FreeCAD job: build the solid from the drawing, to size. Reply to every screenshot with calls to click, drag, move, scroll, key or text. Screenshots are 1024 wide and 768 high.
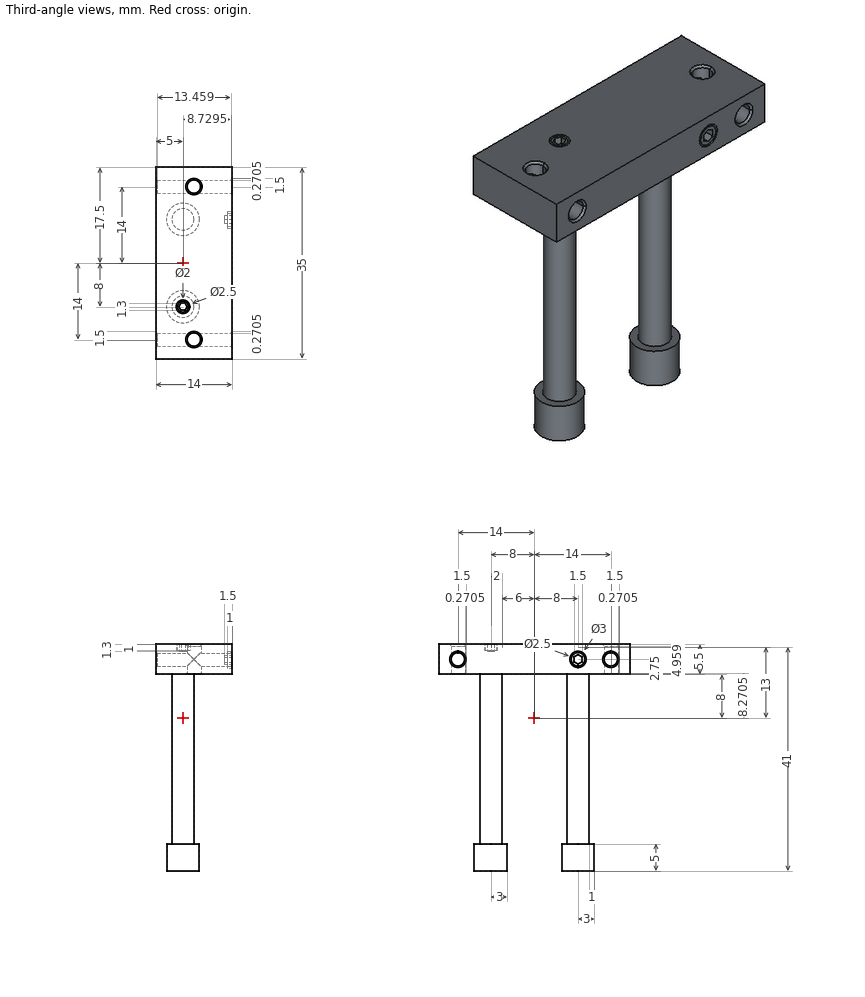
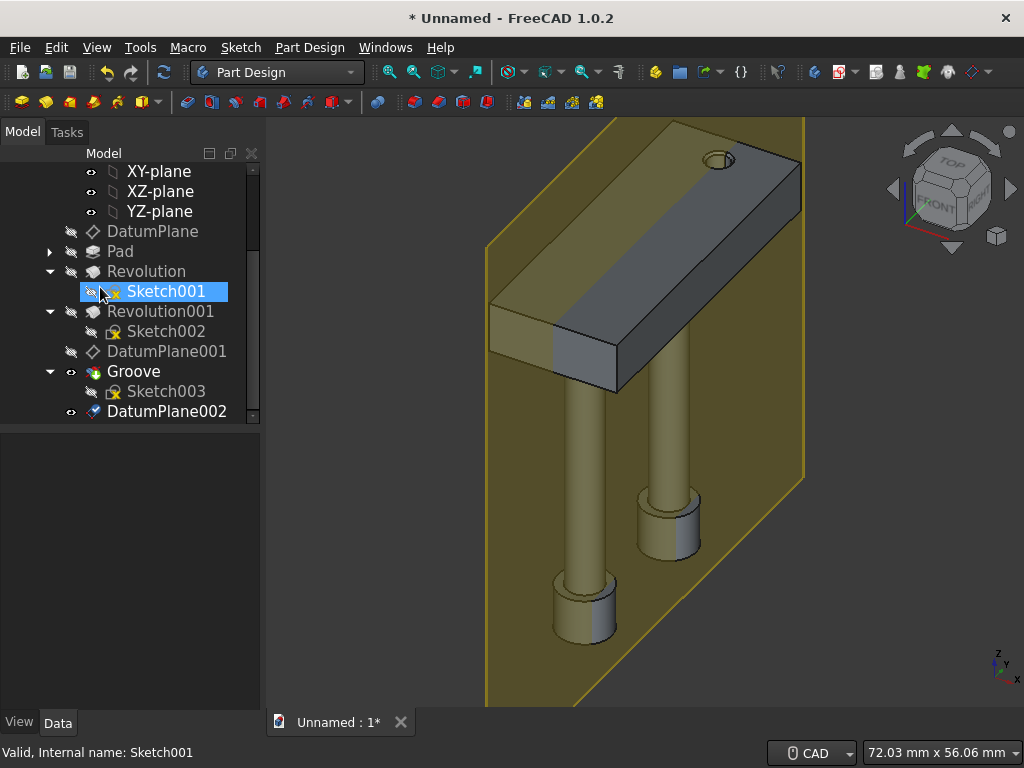
click(116, 412)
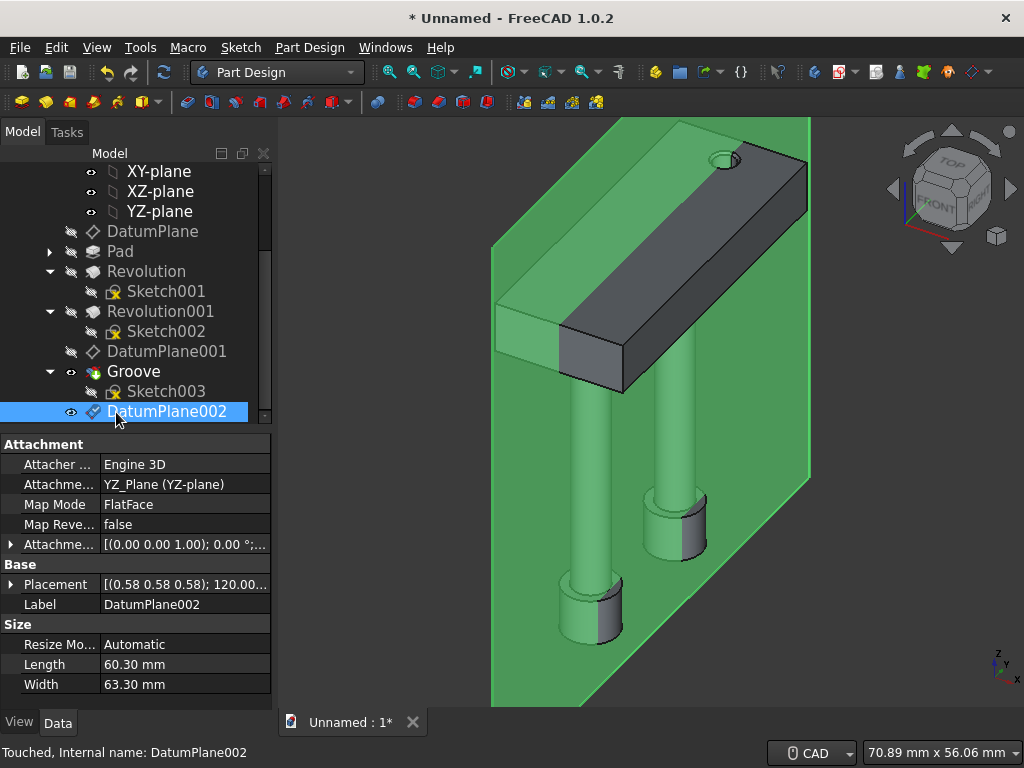
click(840, 72)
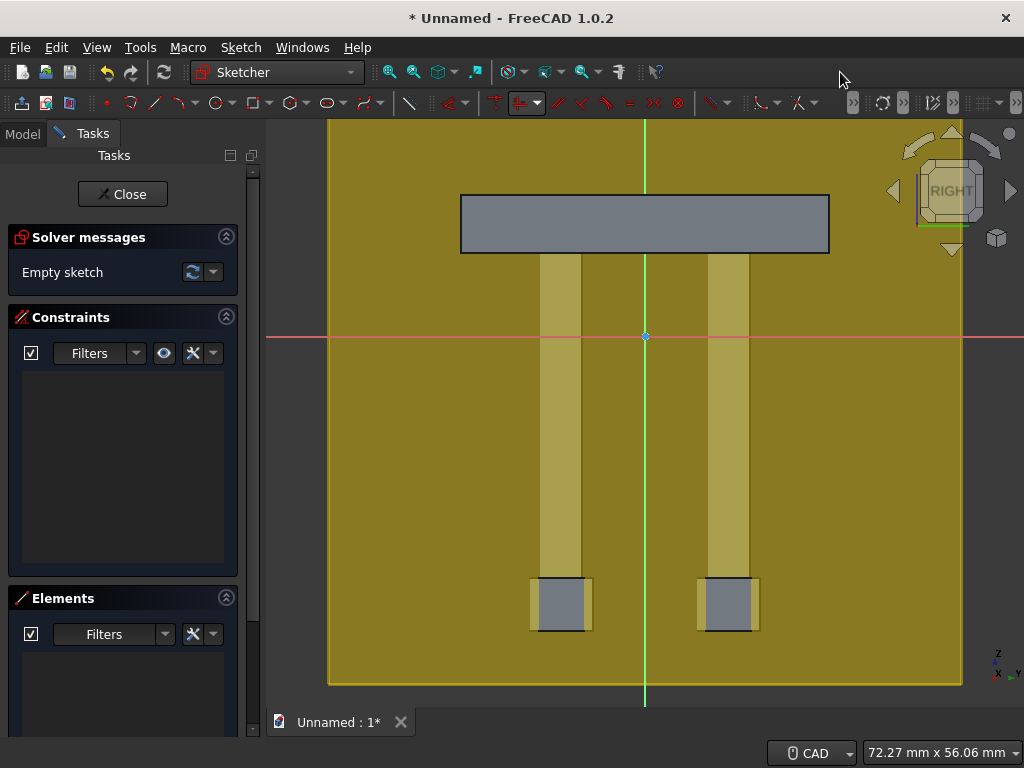
click(70, 104)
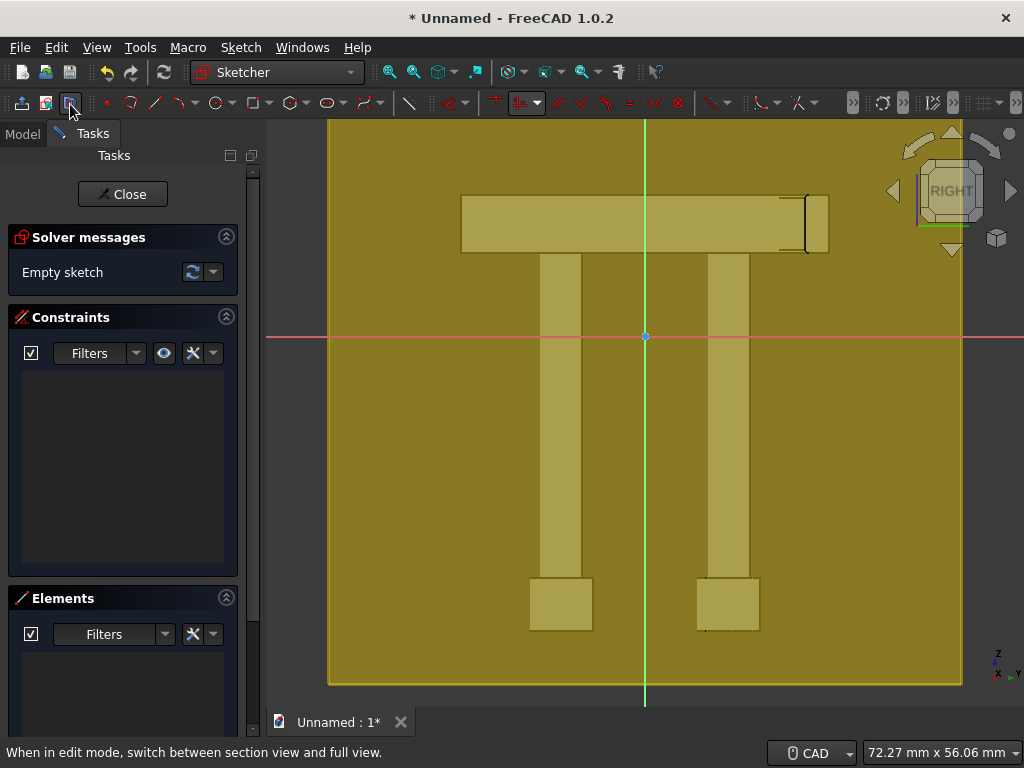
scroll(568, 147, up, 4)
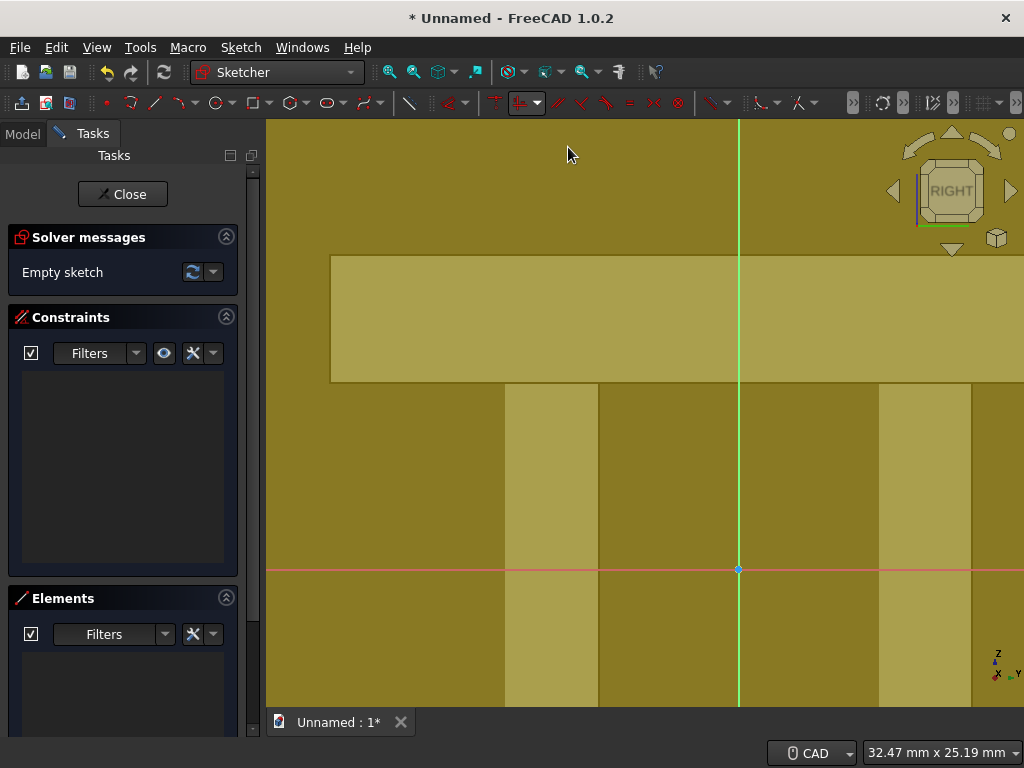
click(132, 104)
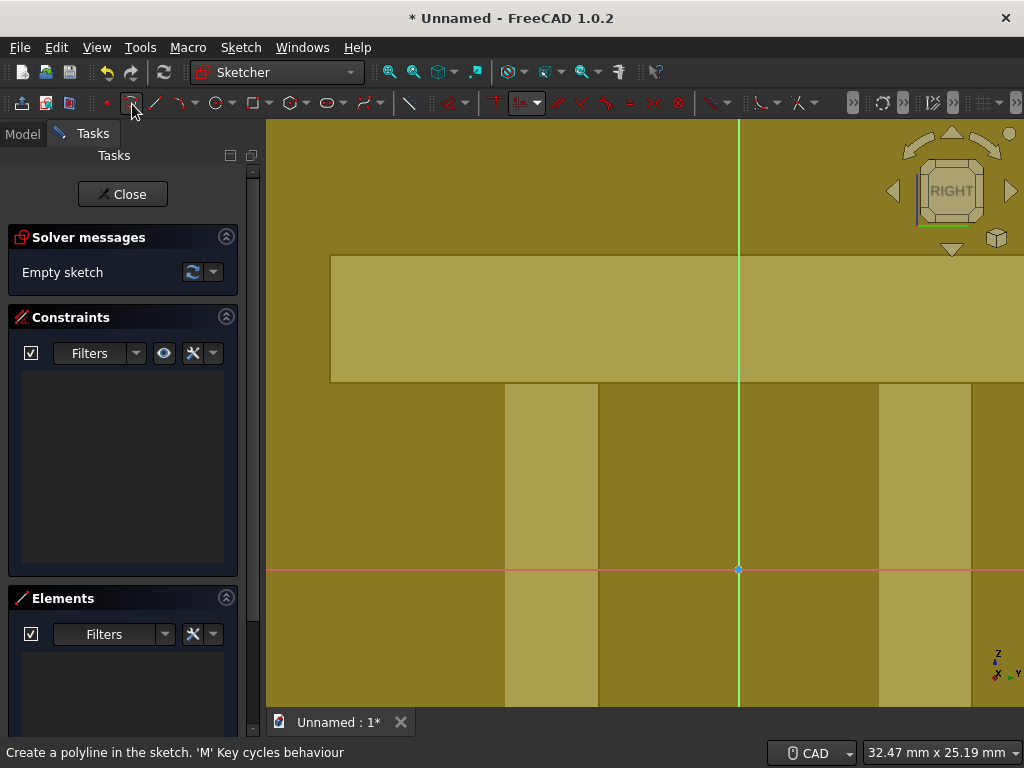
click(447, 383)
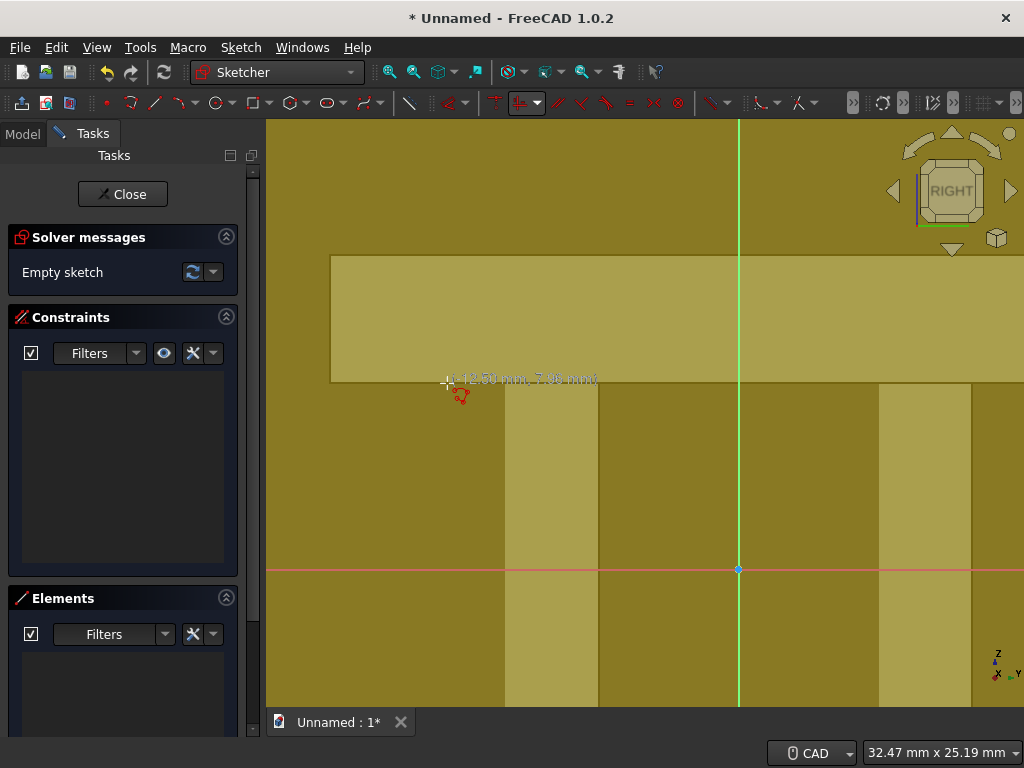
scroll(441, 377, up, 3)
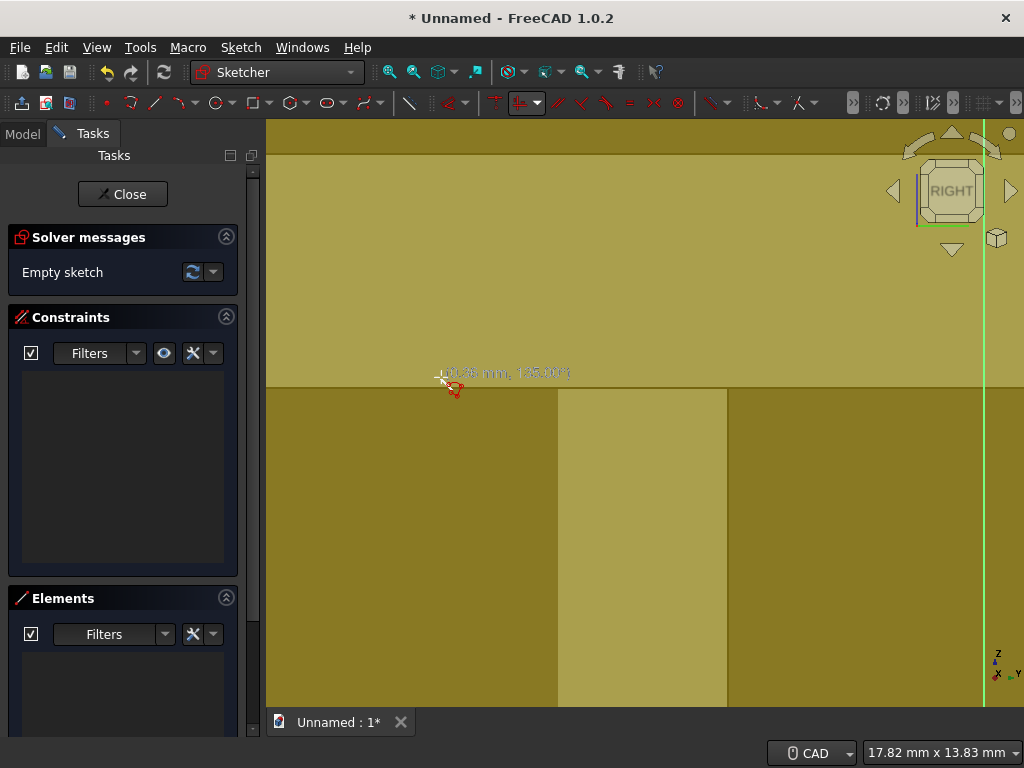
click(440, 376)
click(440, 165)
click(452, 154)
click(388, 154)
click(388, 388)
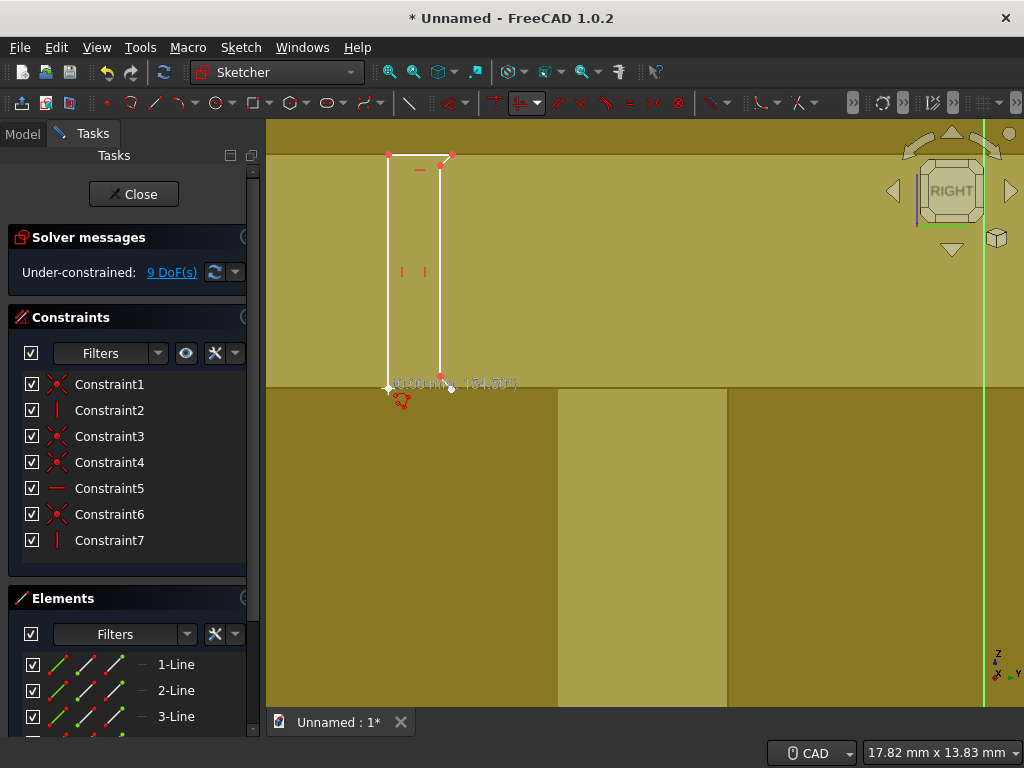
scroll(452, 388, up, 4)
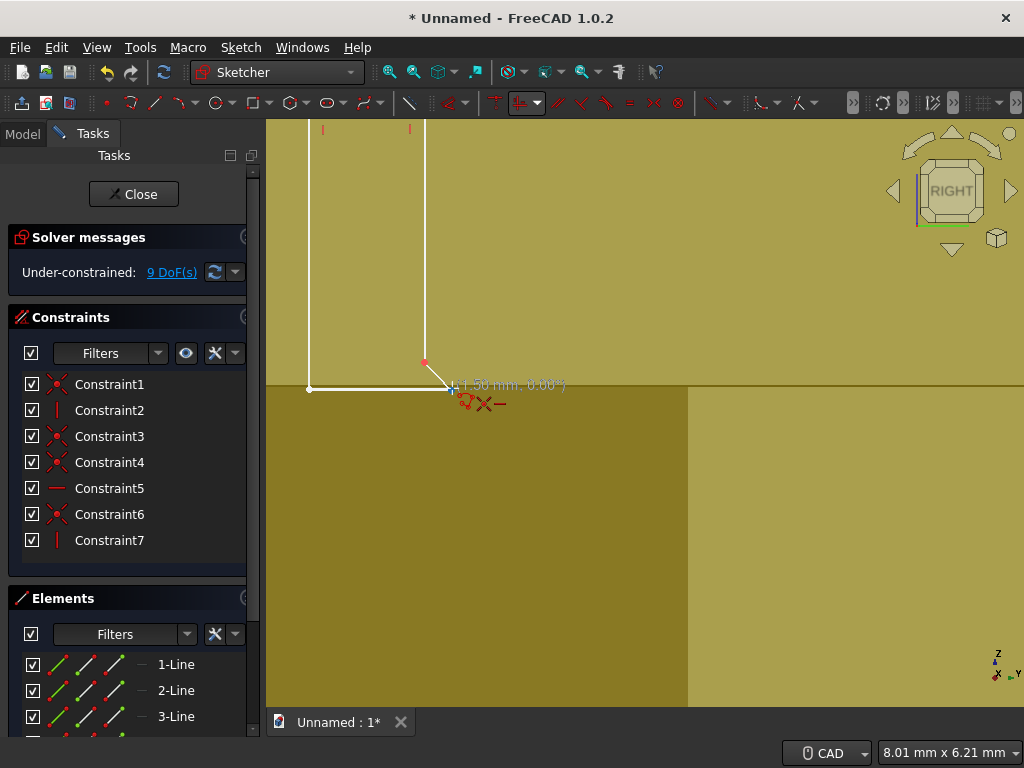
click(451, 391)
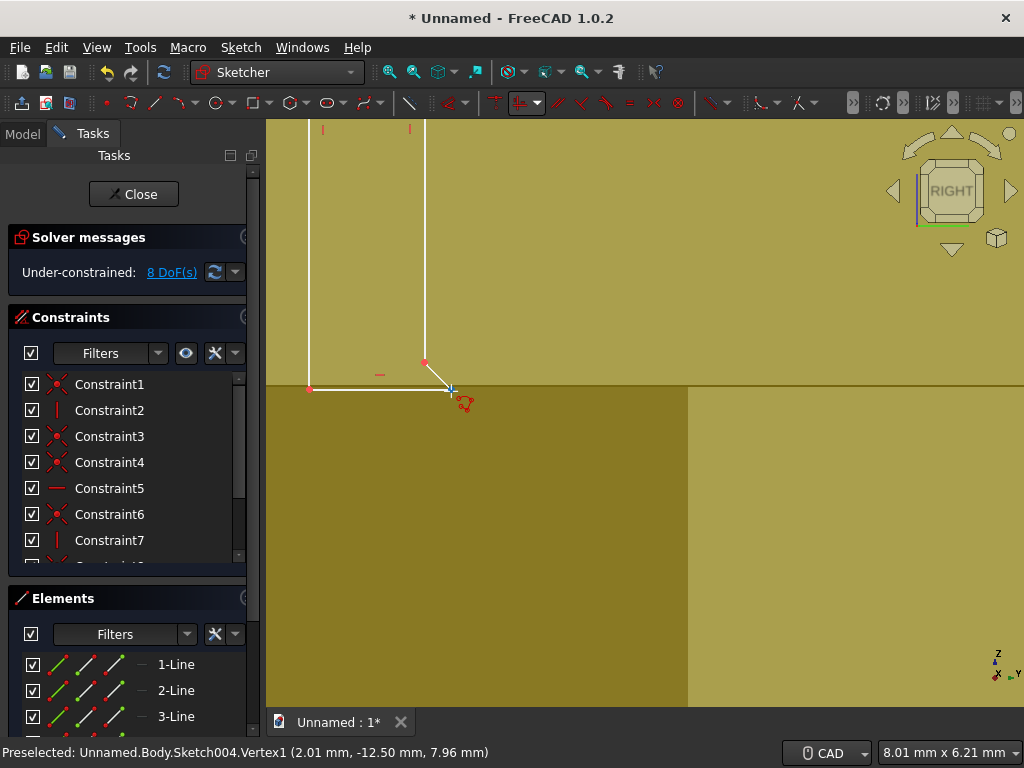
click(156, 104)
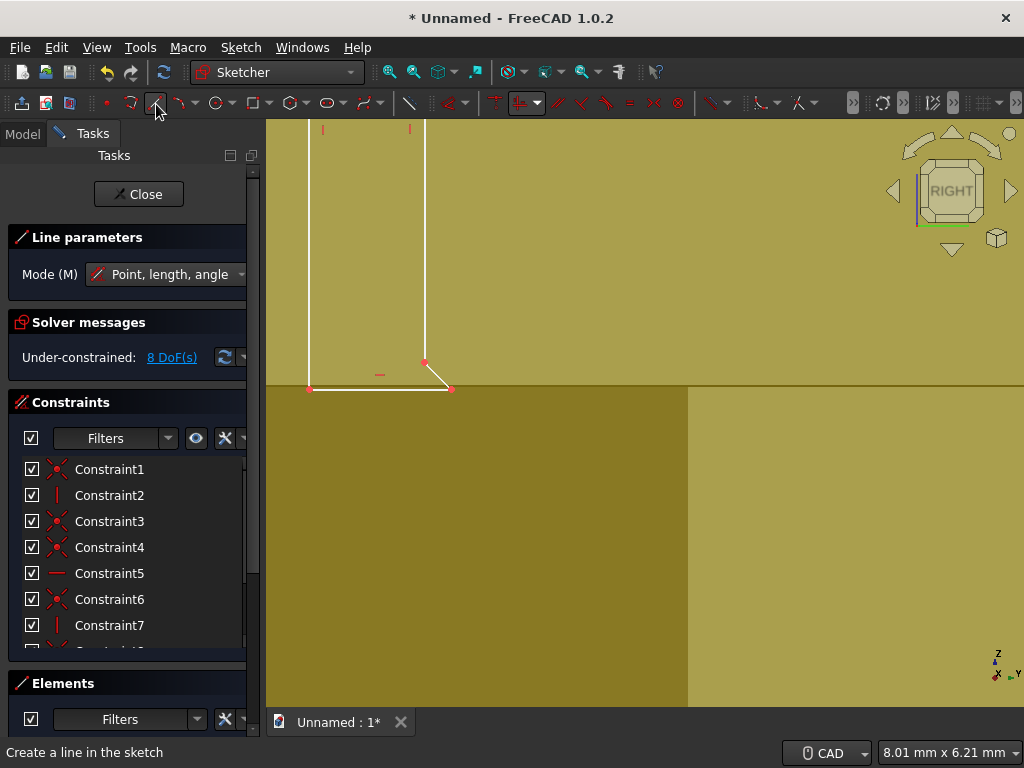
scroll(447, 417, down, 7)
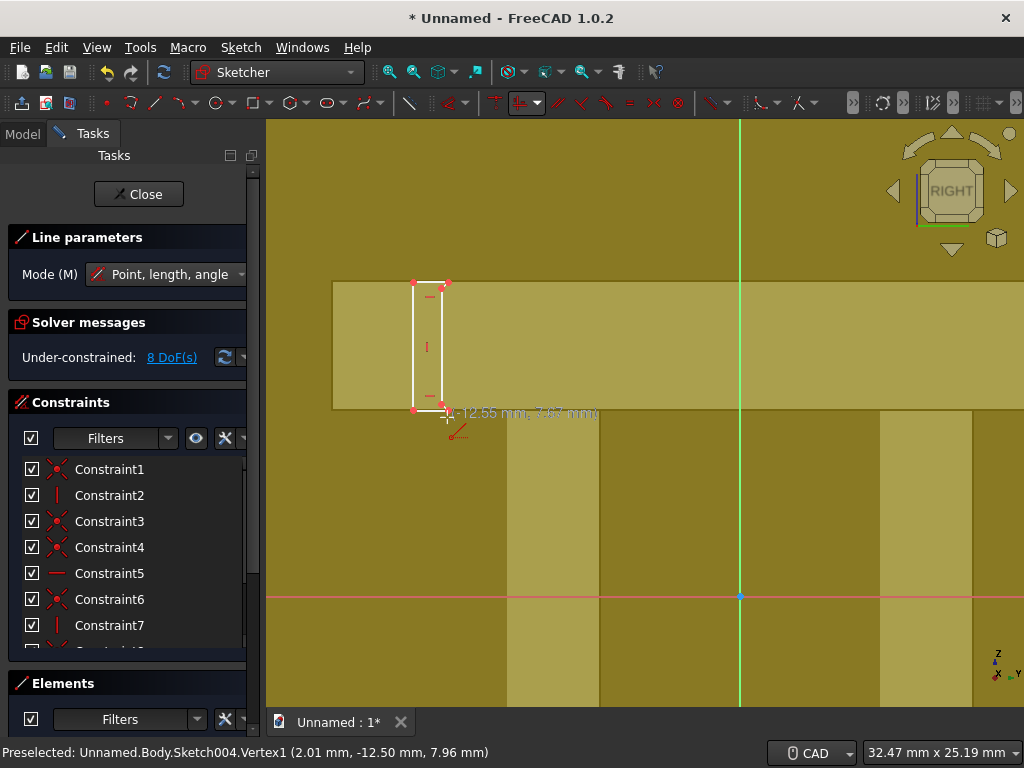
scroll(413, 269, up, 2)